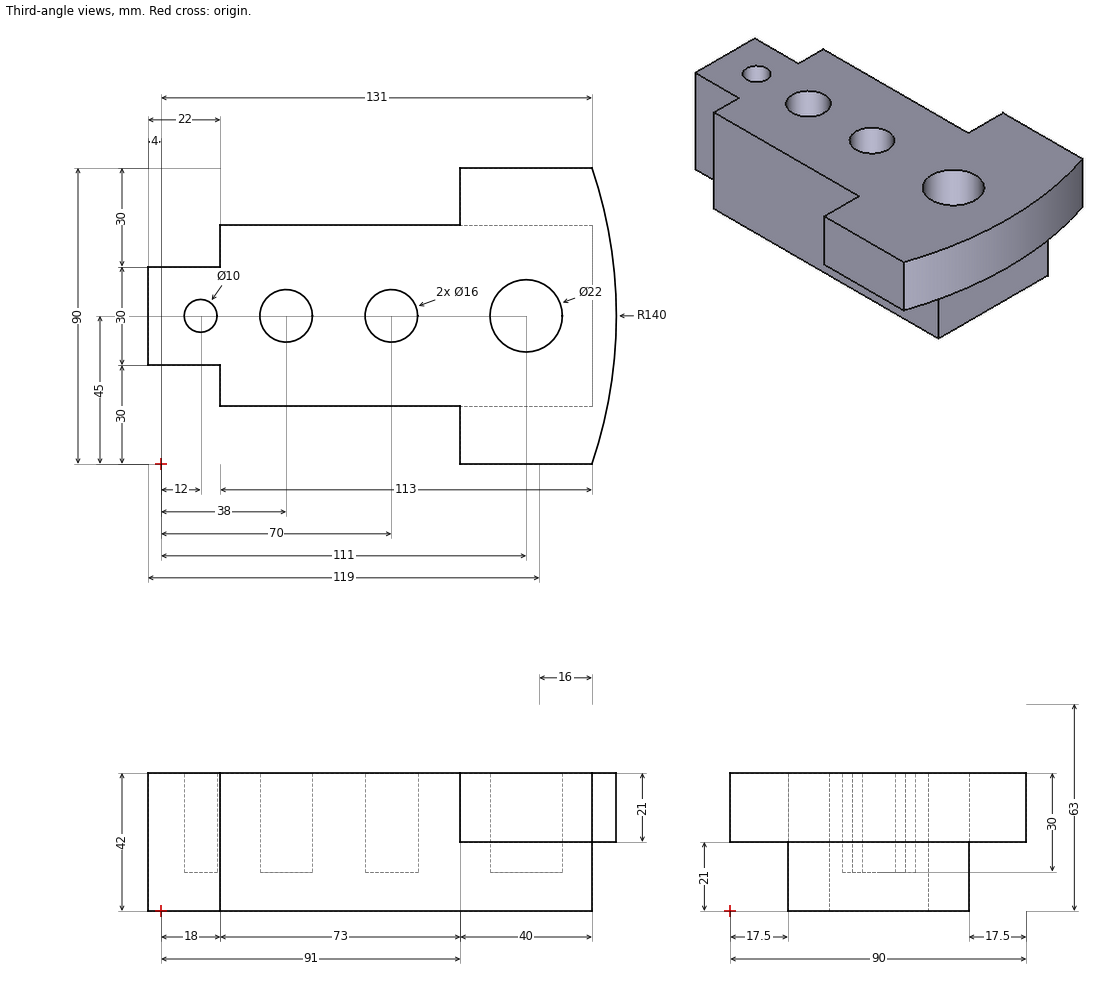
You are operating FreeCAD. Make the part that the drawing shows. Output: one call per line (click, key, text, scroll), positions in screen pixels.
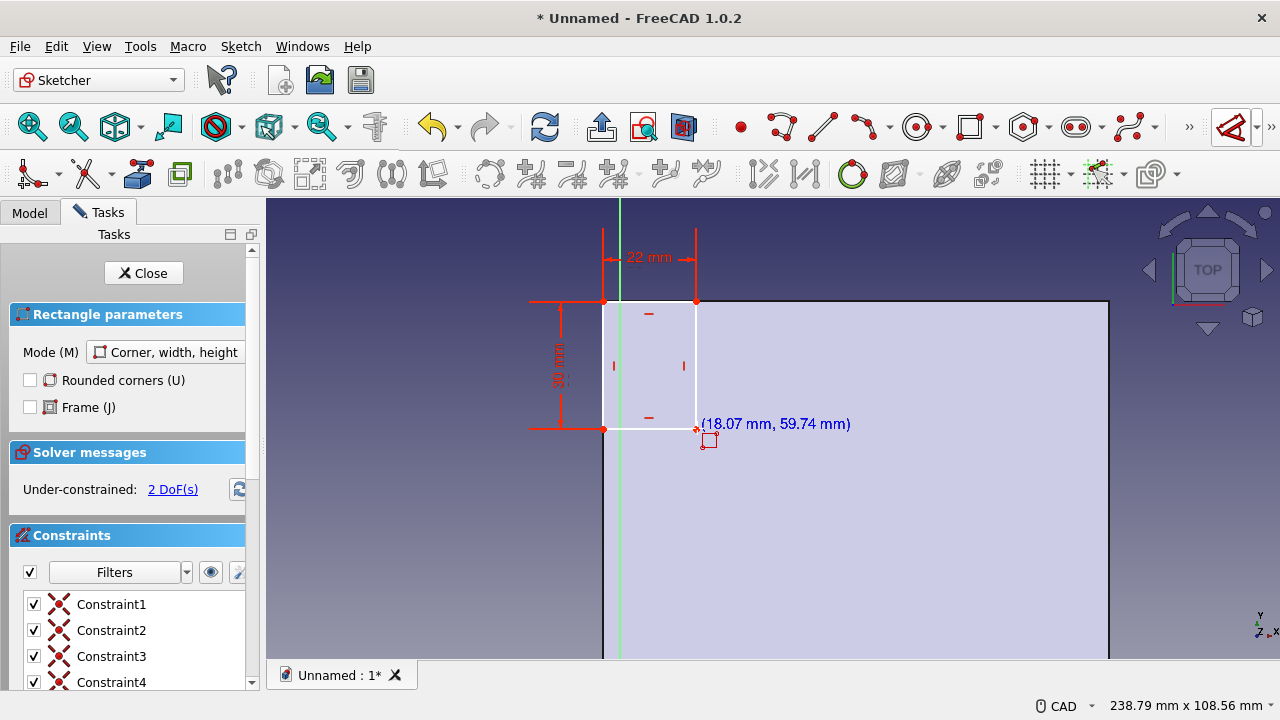
click(603, 555)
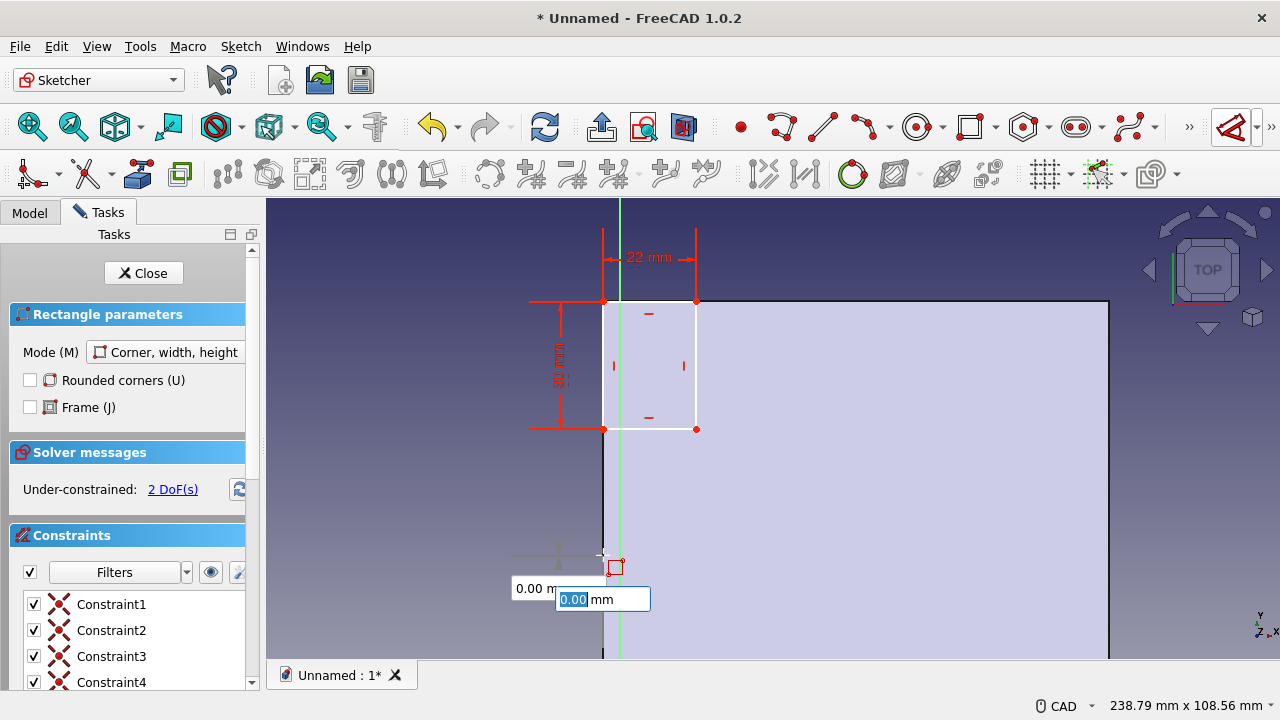
scroll(951, 226, down, 1)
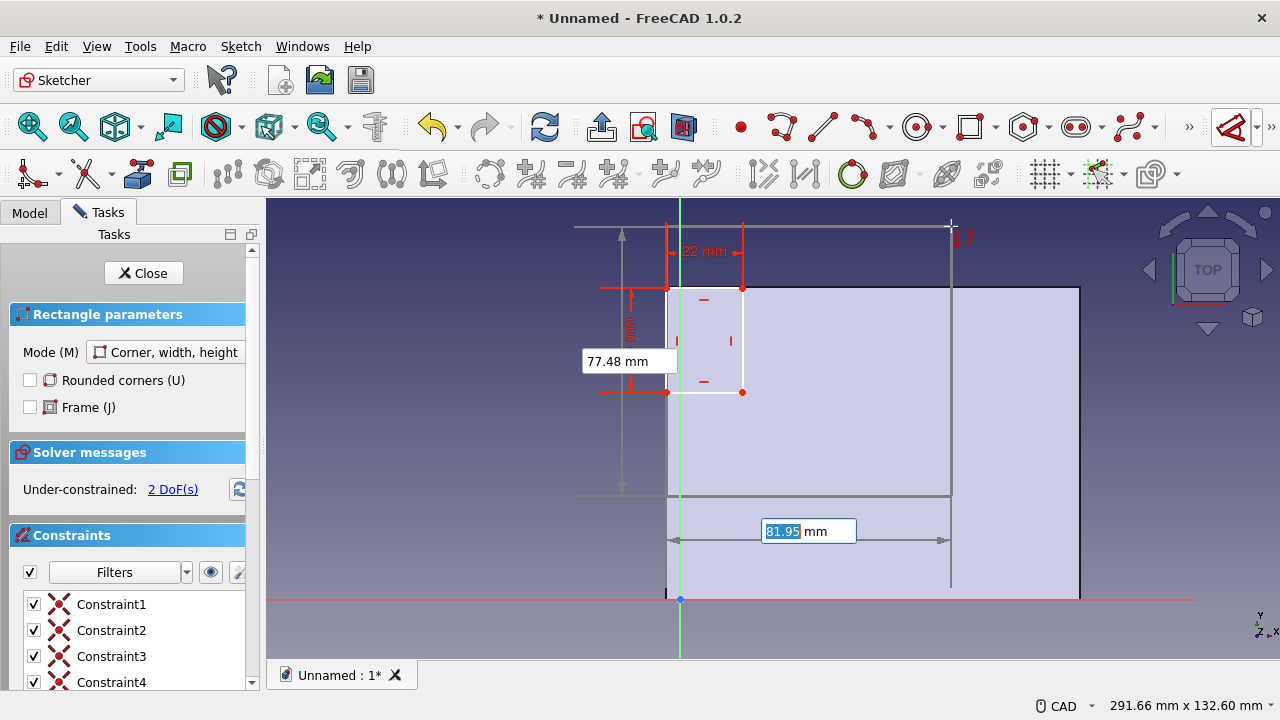
click(743, 600)
key(Escape)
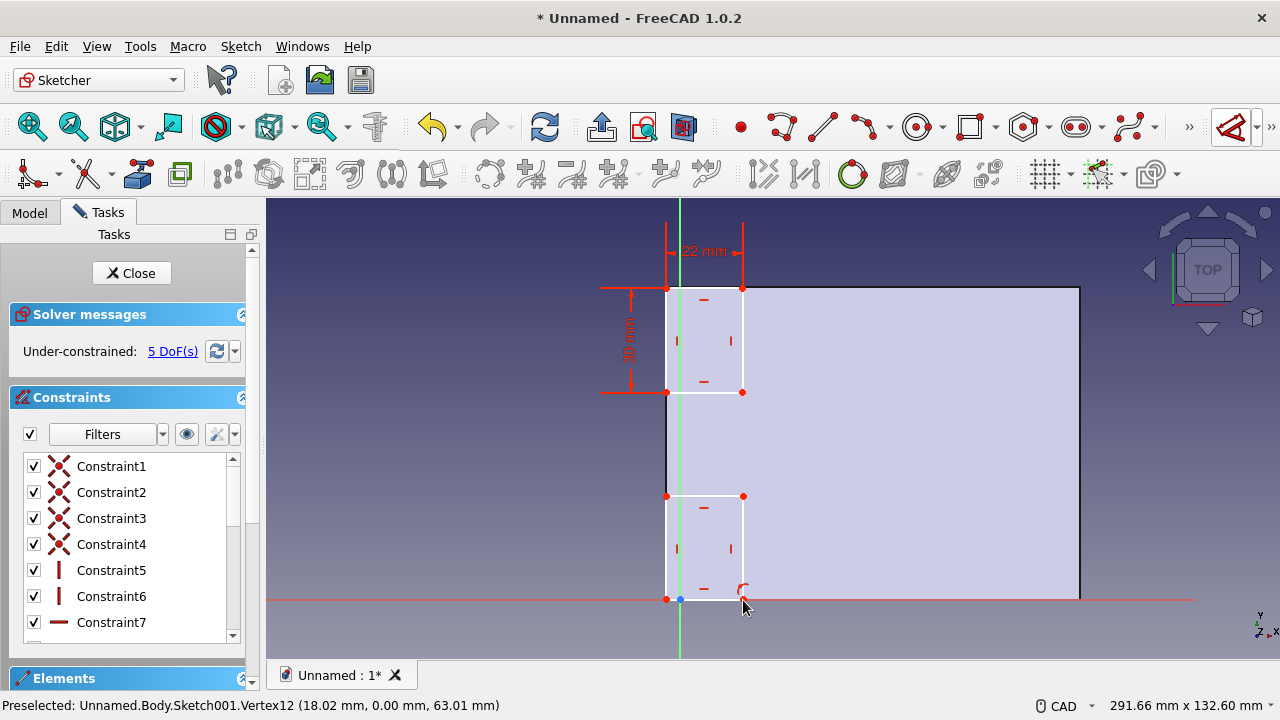
click(666, 527)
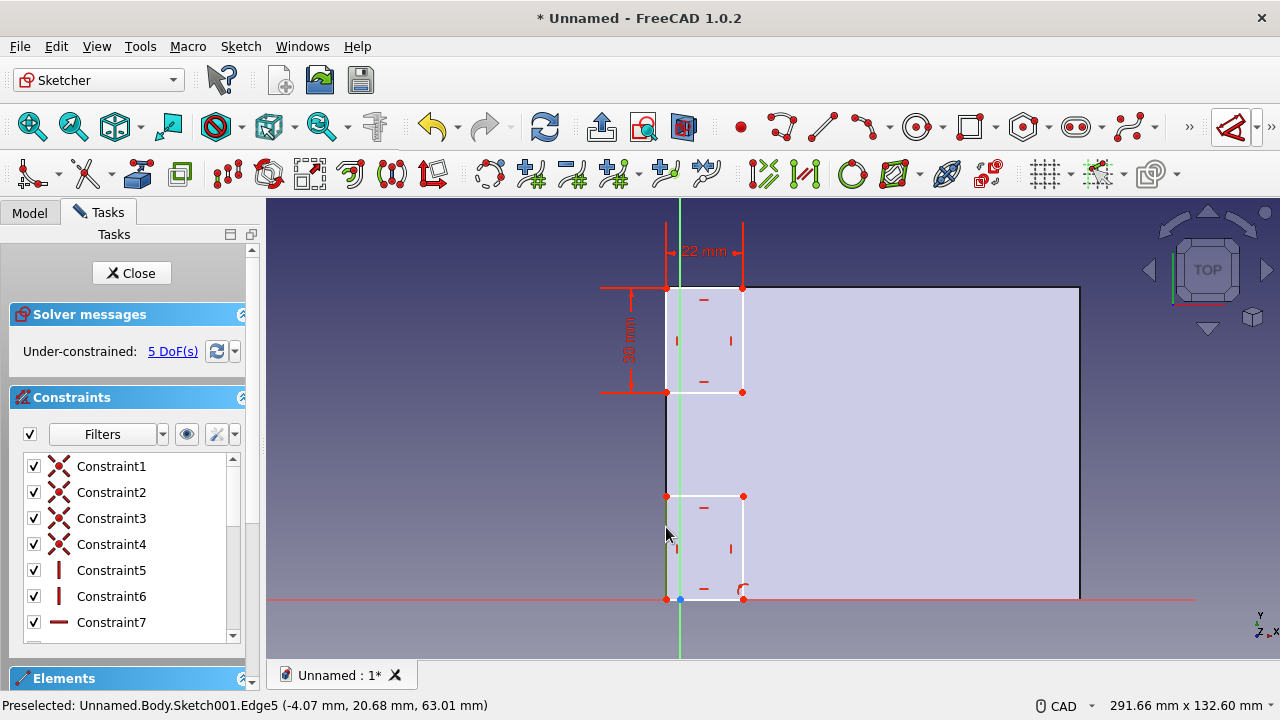
click(1256, 128)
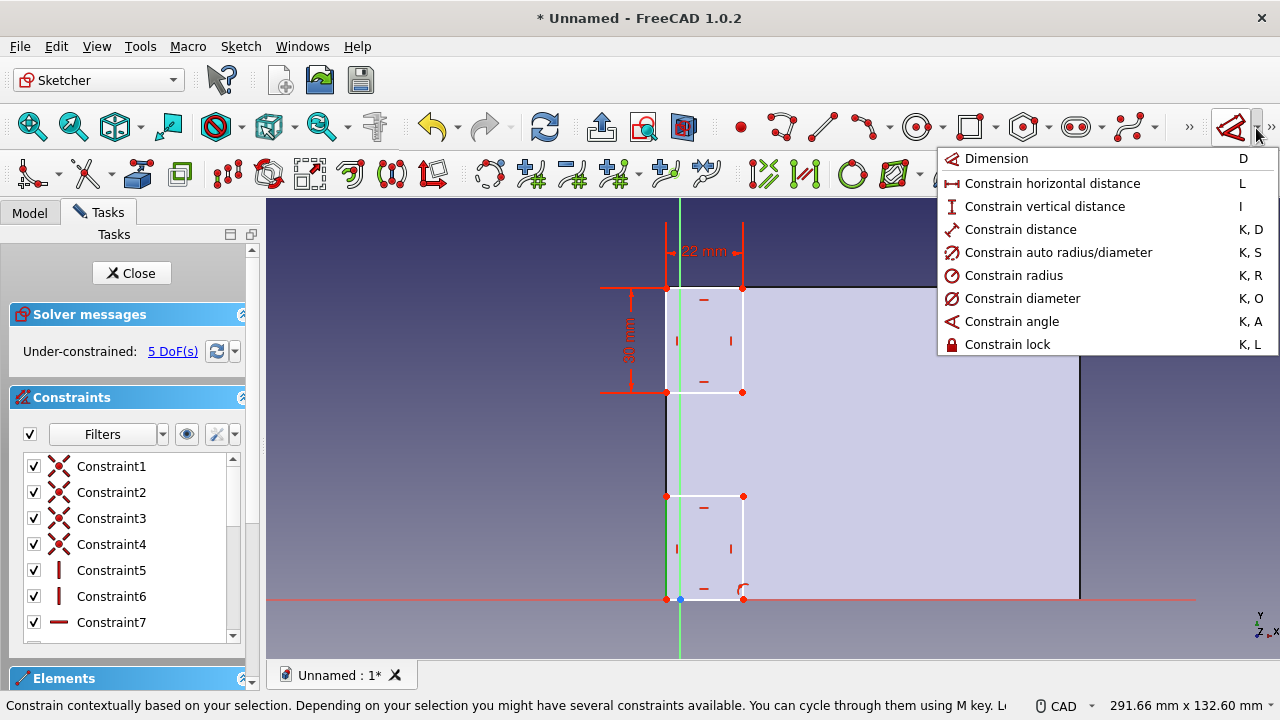
click(1108, 206)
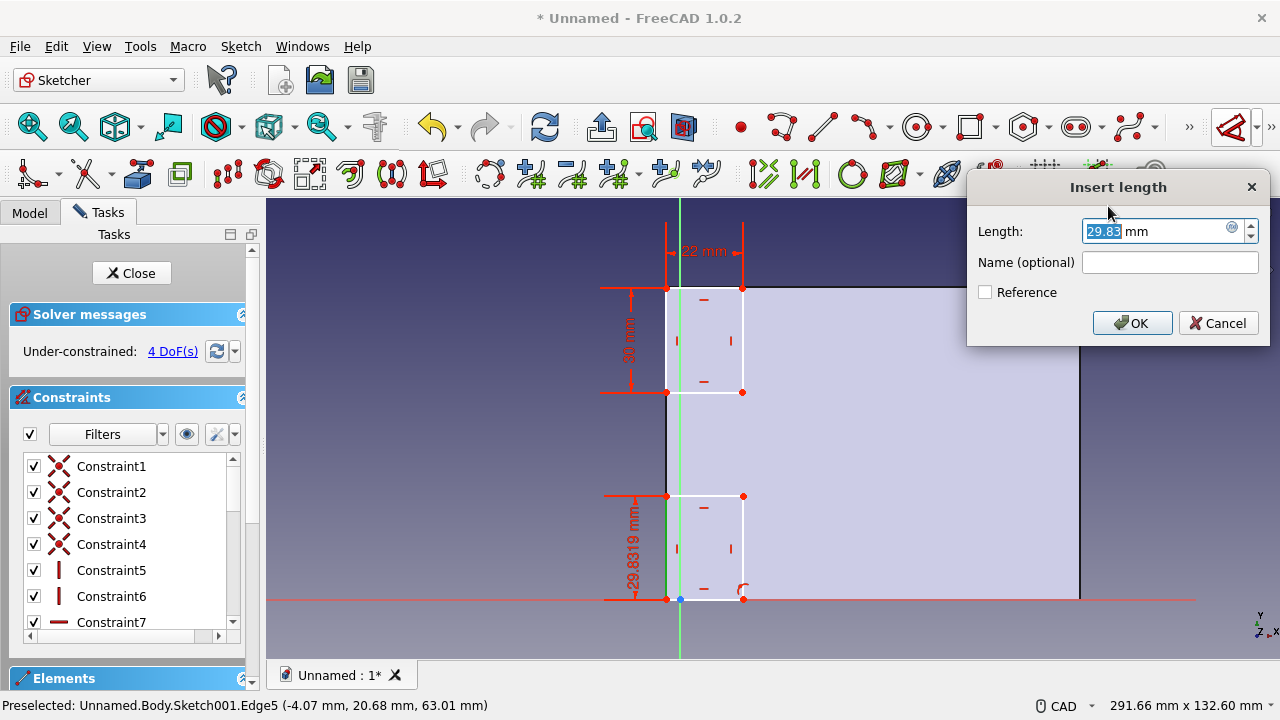
text(30)
key(Return)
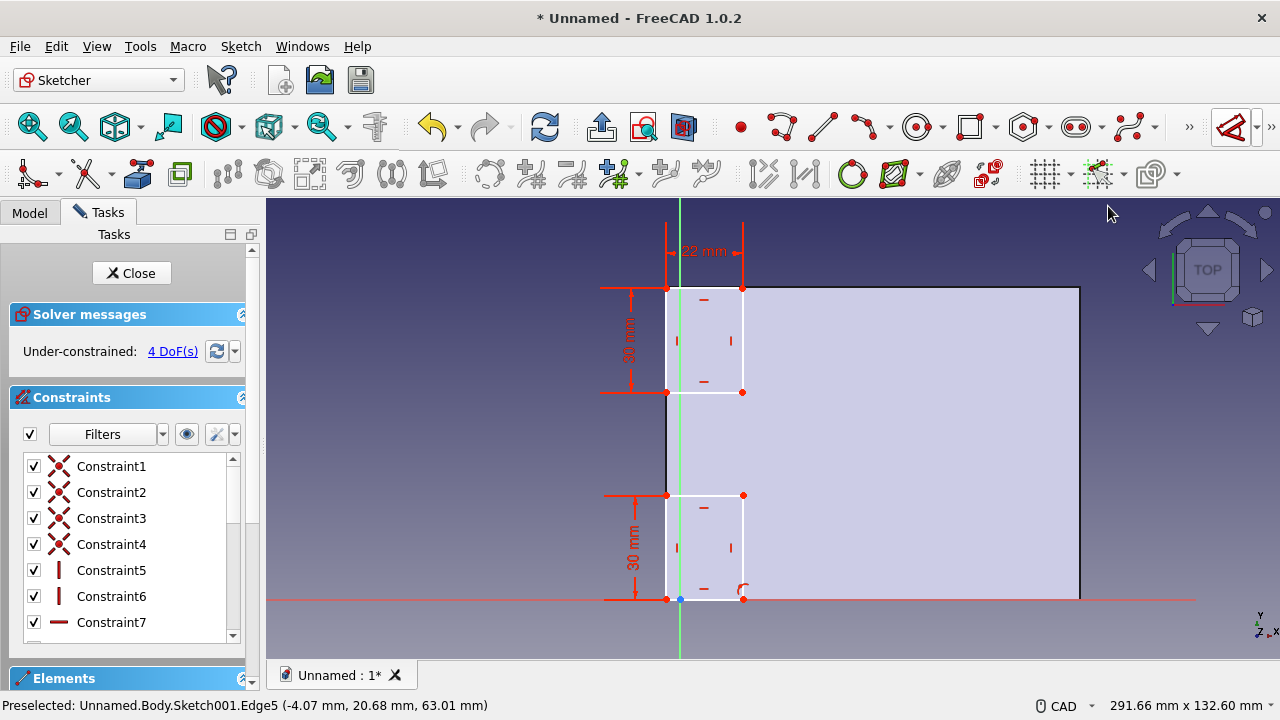
click(720, 600)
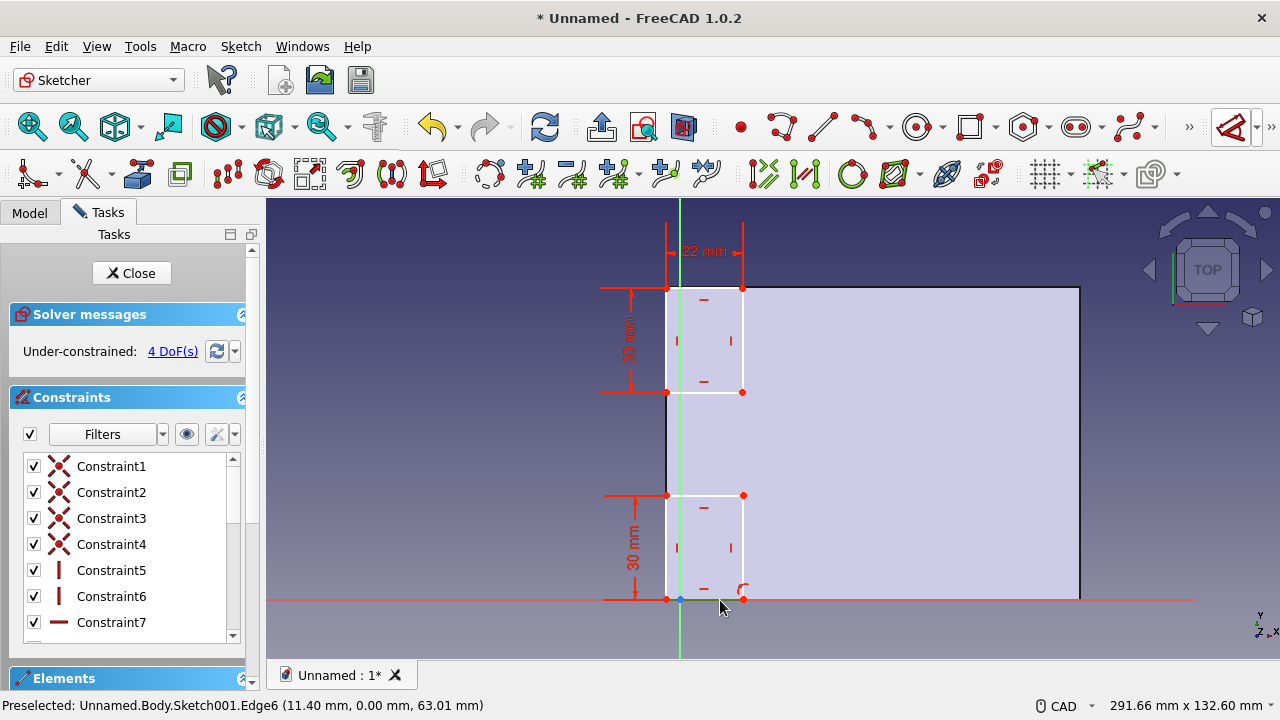
click(1256, 128)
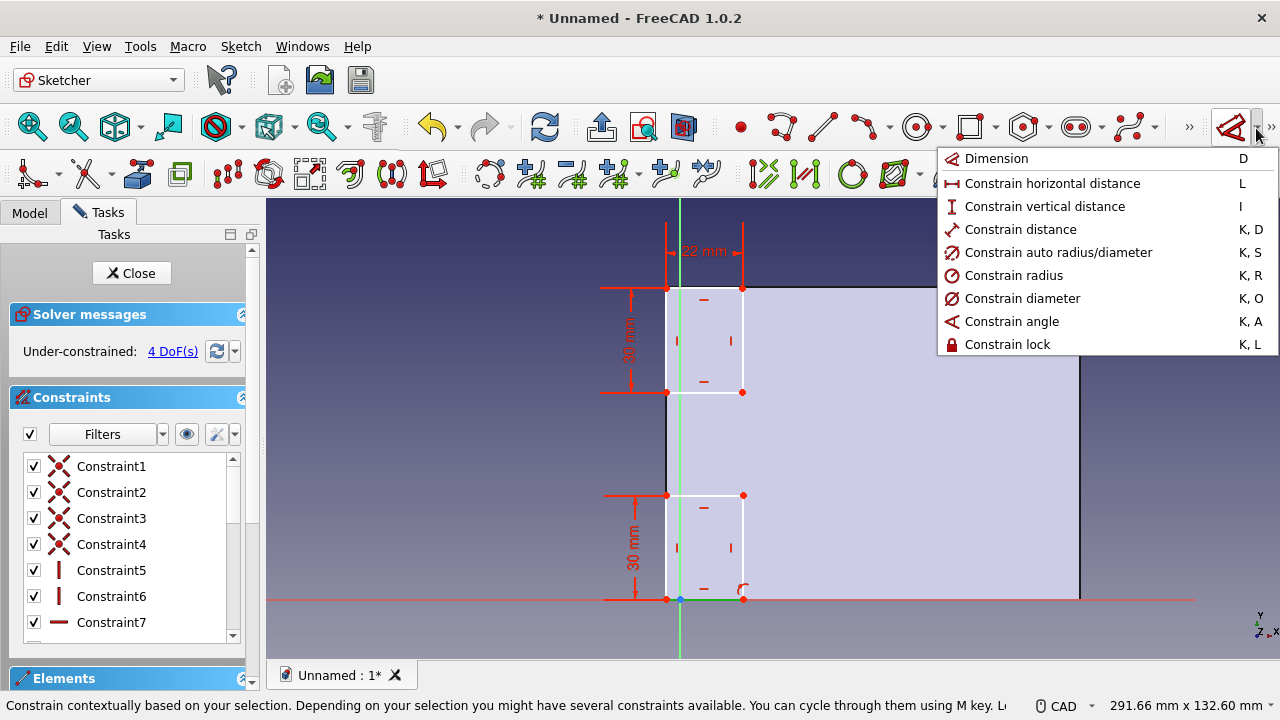
click(1108, 184)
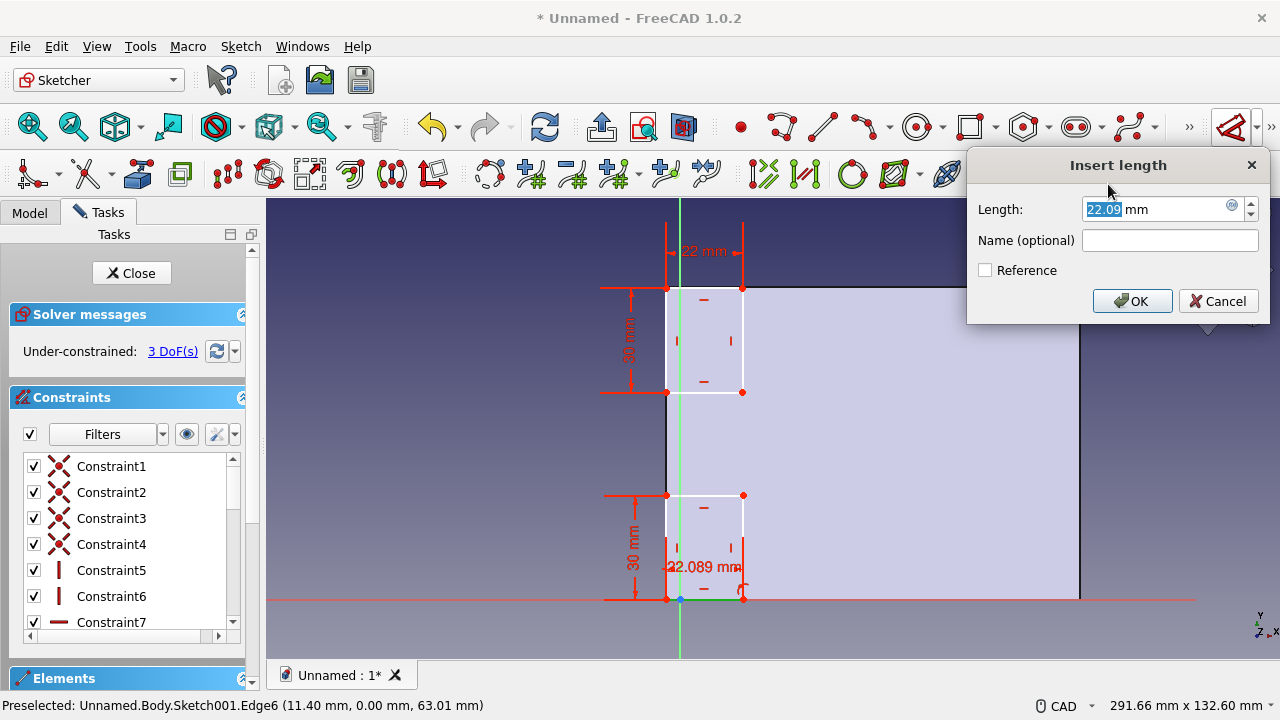
text(22)
key(Return)